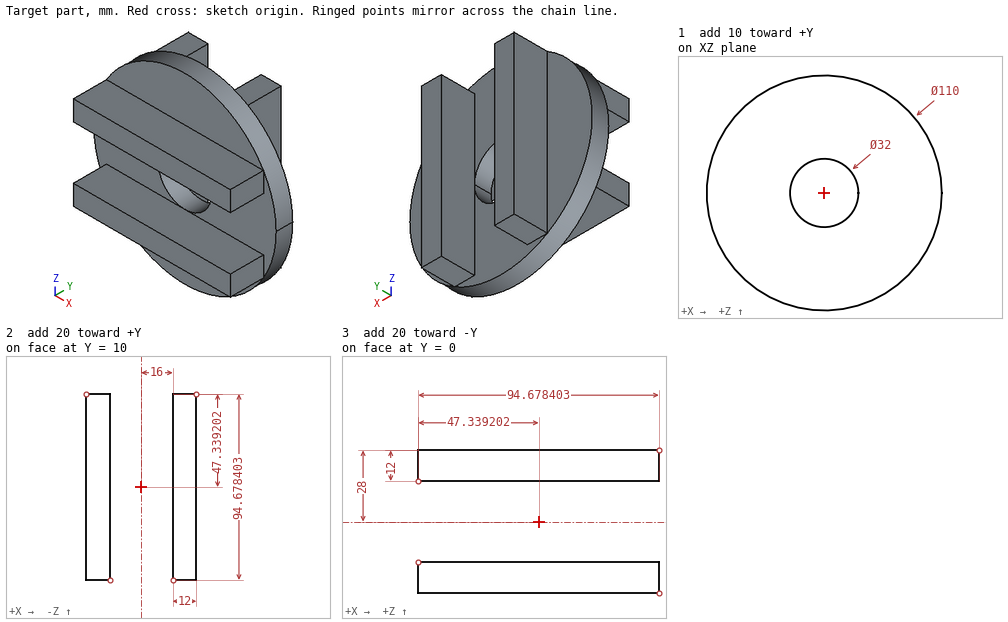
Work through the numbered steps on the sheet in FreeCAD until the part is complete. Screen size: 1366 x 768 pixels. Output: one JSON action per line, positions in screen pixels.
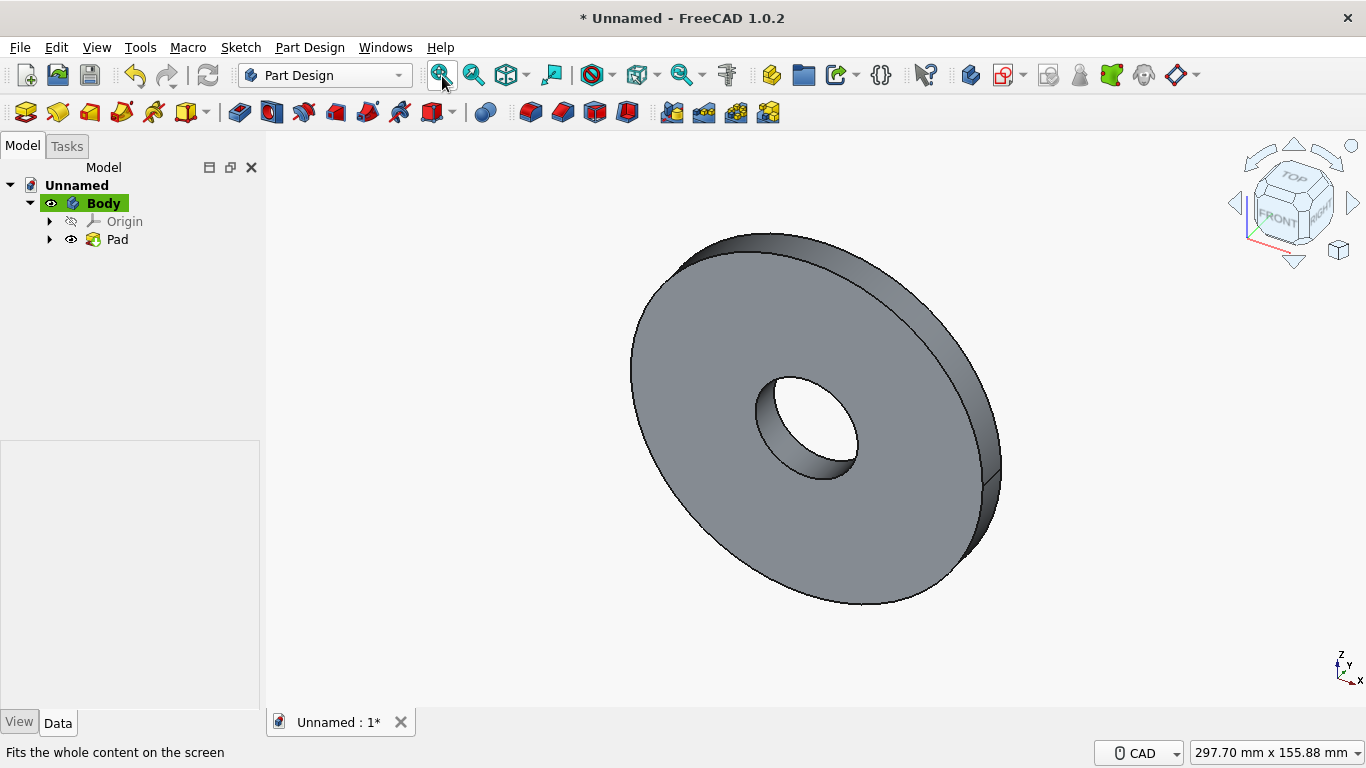
{"action": "key", "text": "4"}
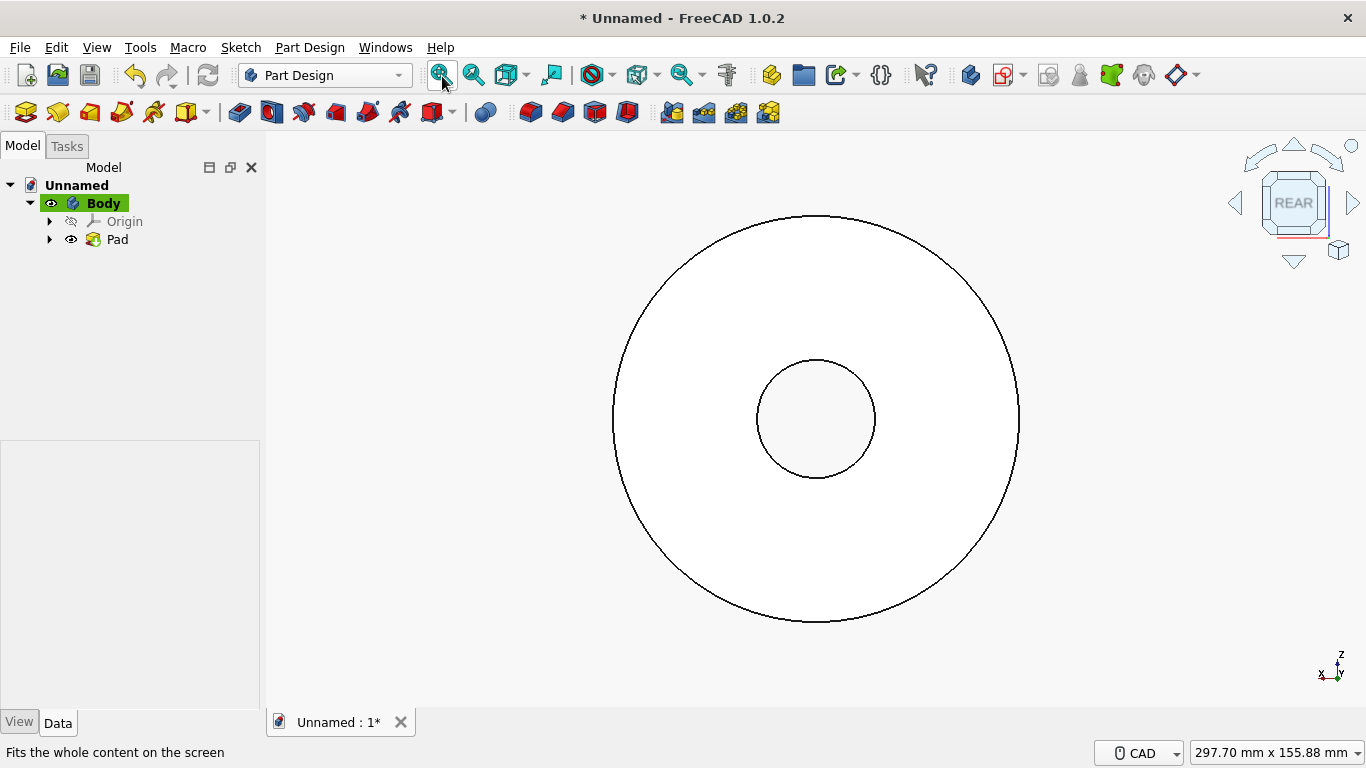
{"action": "left_click", "coordinate": [874, 302]}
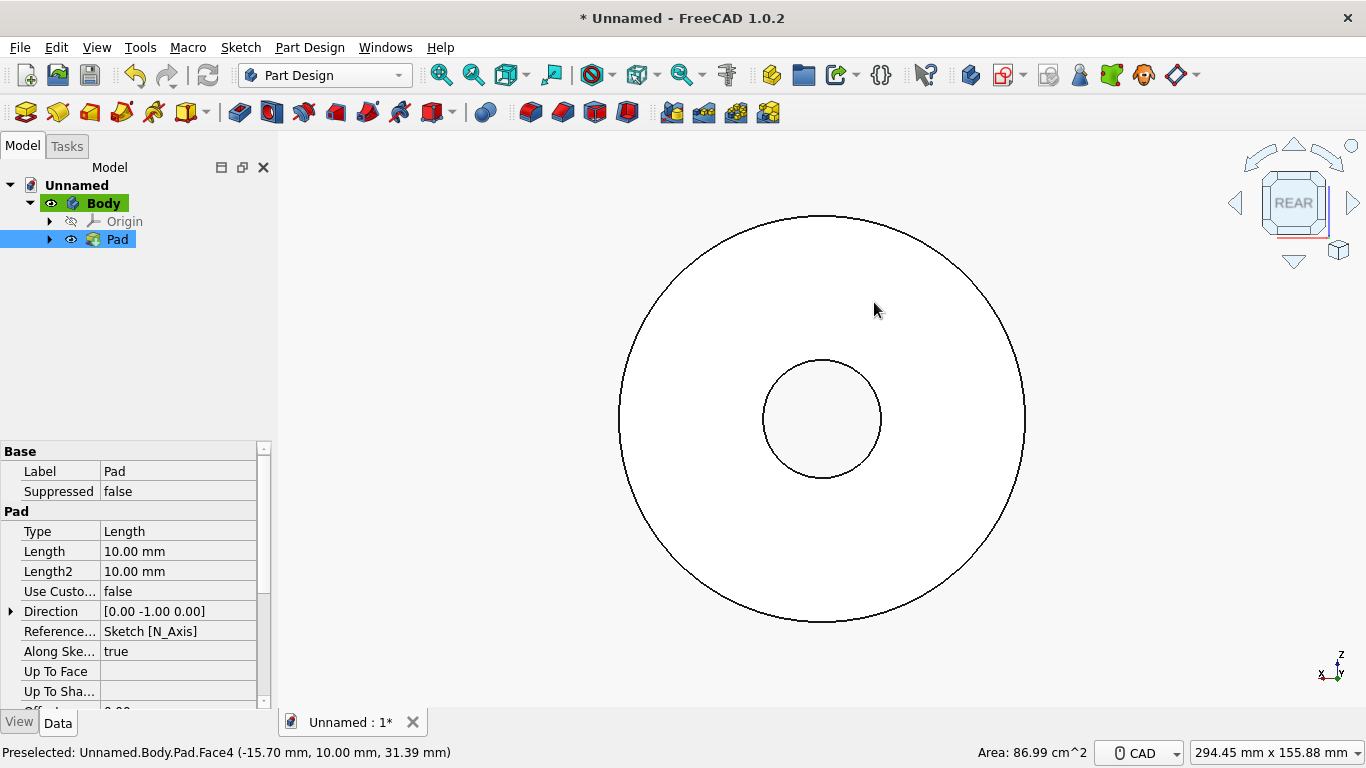
{"action": "left_click", "coordinate": [1004, 76]}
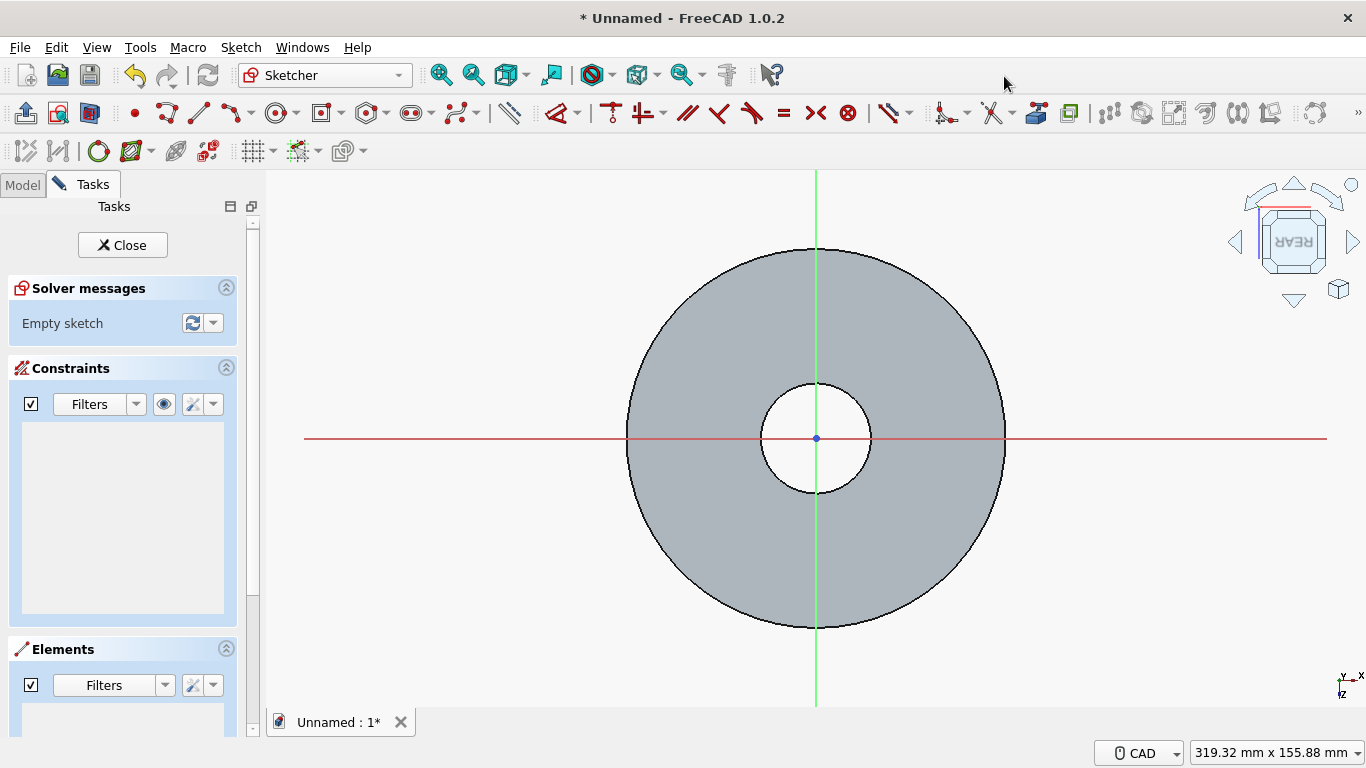
{"action": "key", "text": "g r"}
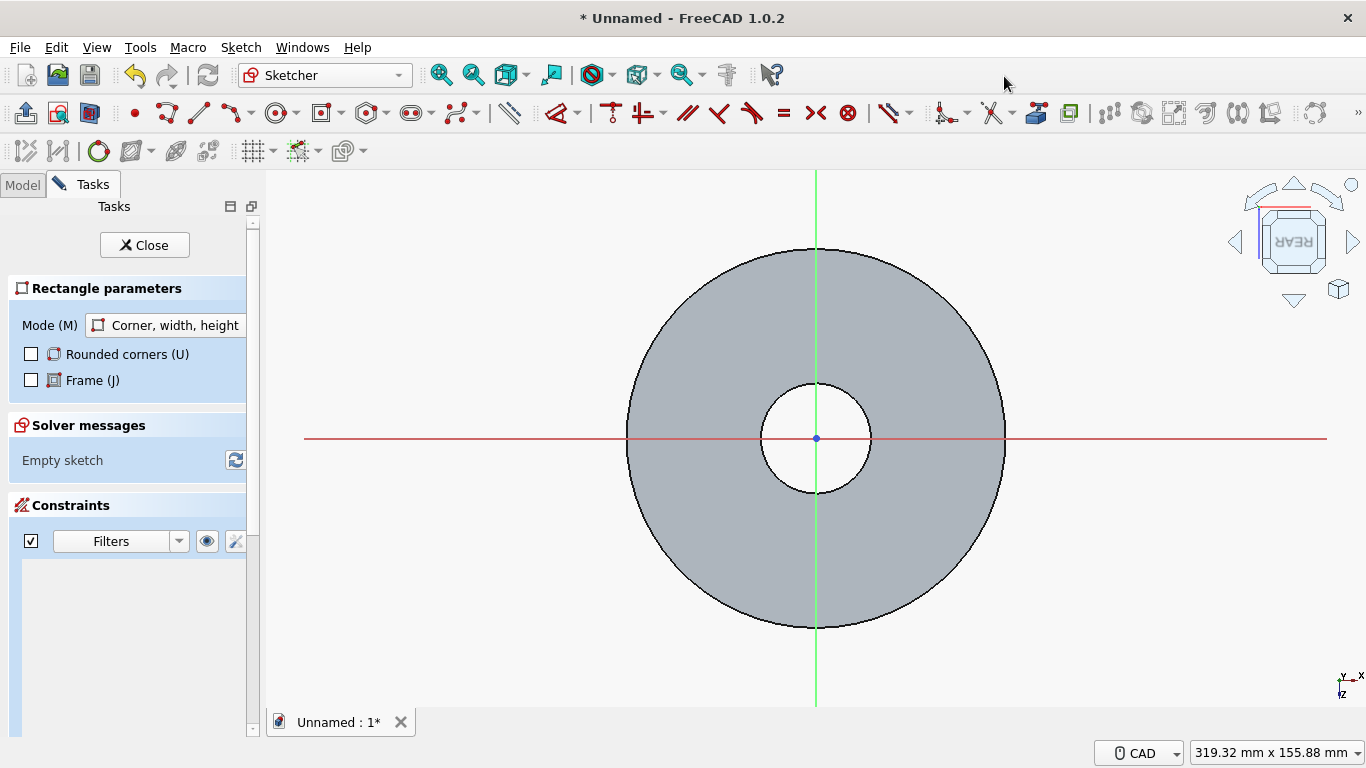
{"action": "left_click", "coordinate": [871, 275]}
{"action": "left_click", "coordinate": [912, 602]}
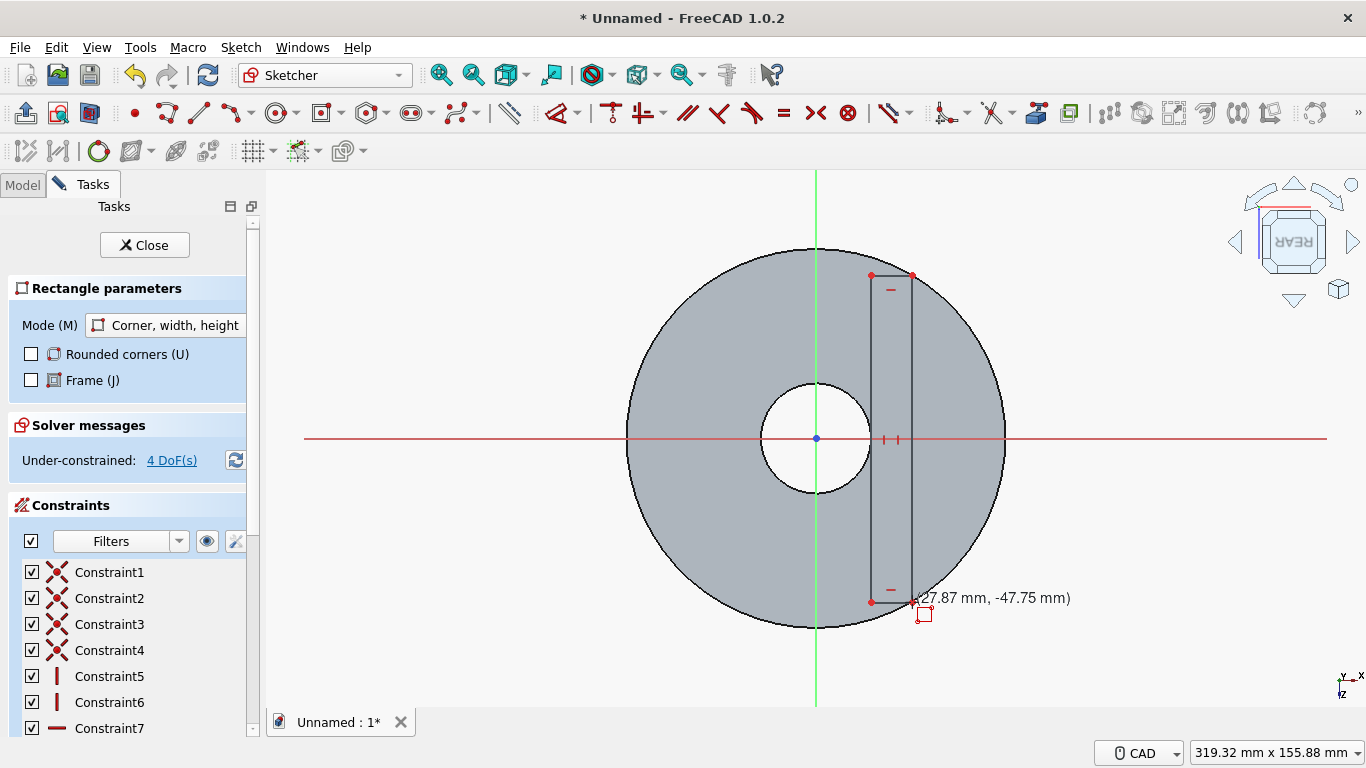
{"action": "left_click", "coordinate": [720, 275]}
{"action": "left_click", "coordinate": [761, 602]}
{"action": "key", "text": "Escape"}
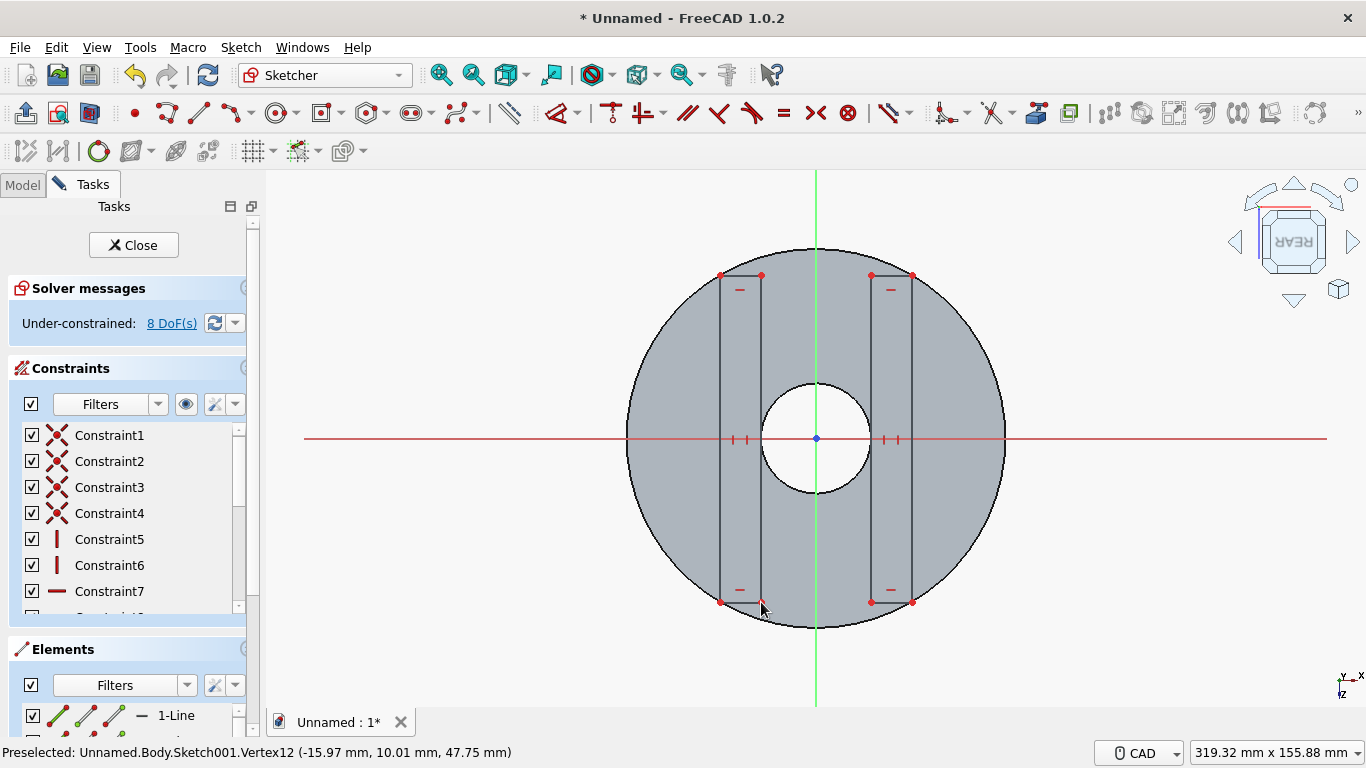
{"action": "left_click", "coordinate": [912, 276]}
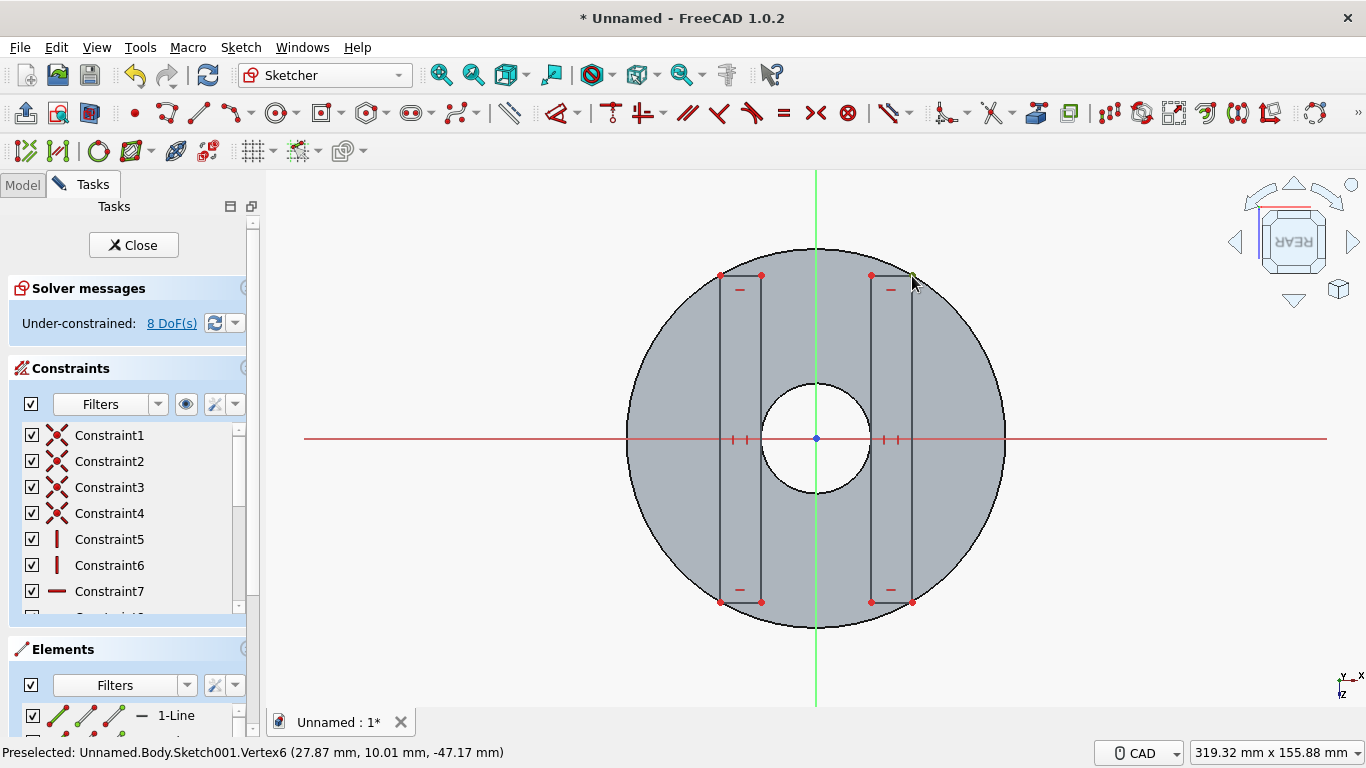
{"action": "left_click", "coordinate": [720, 276]}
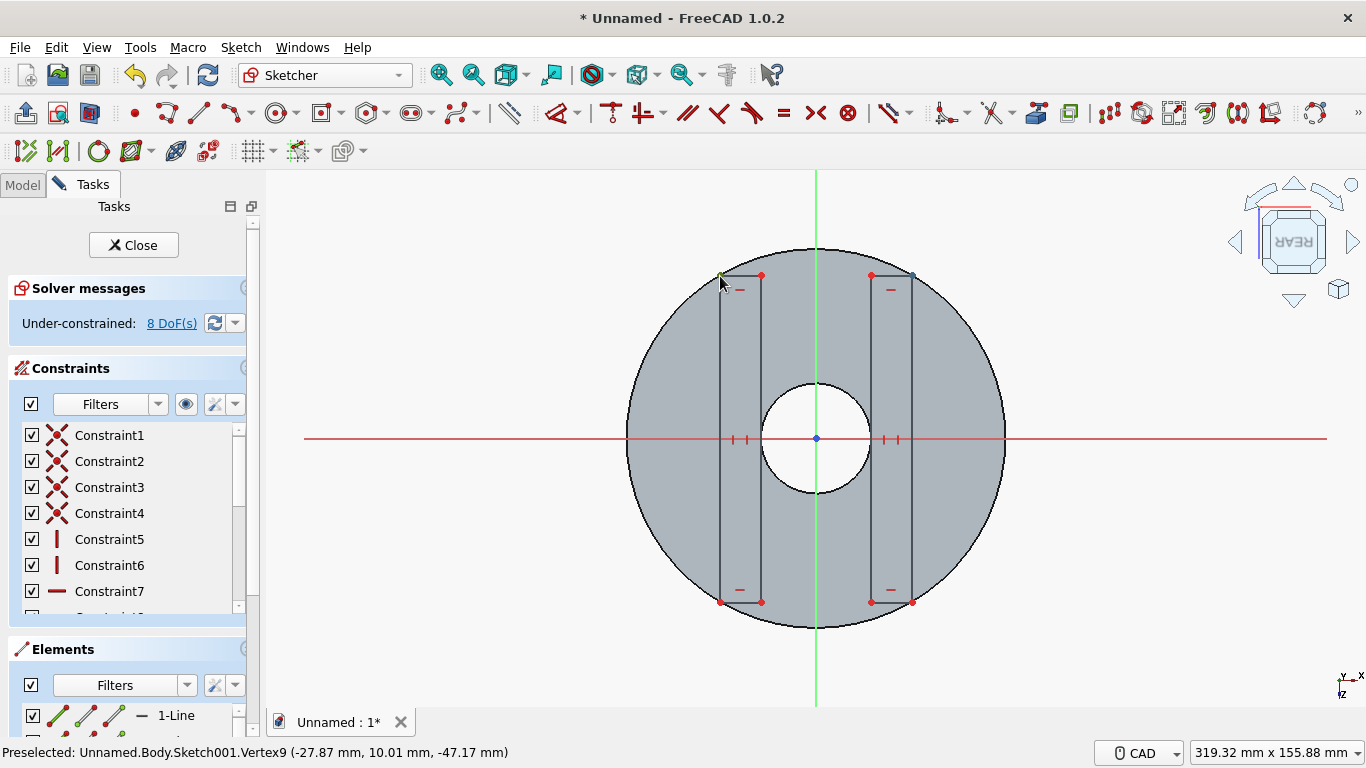
{"action": "left_click", "coordinate": [816, 645]}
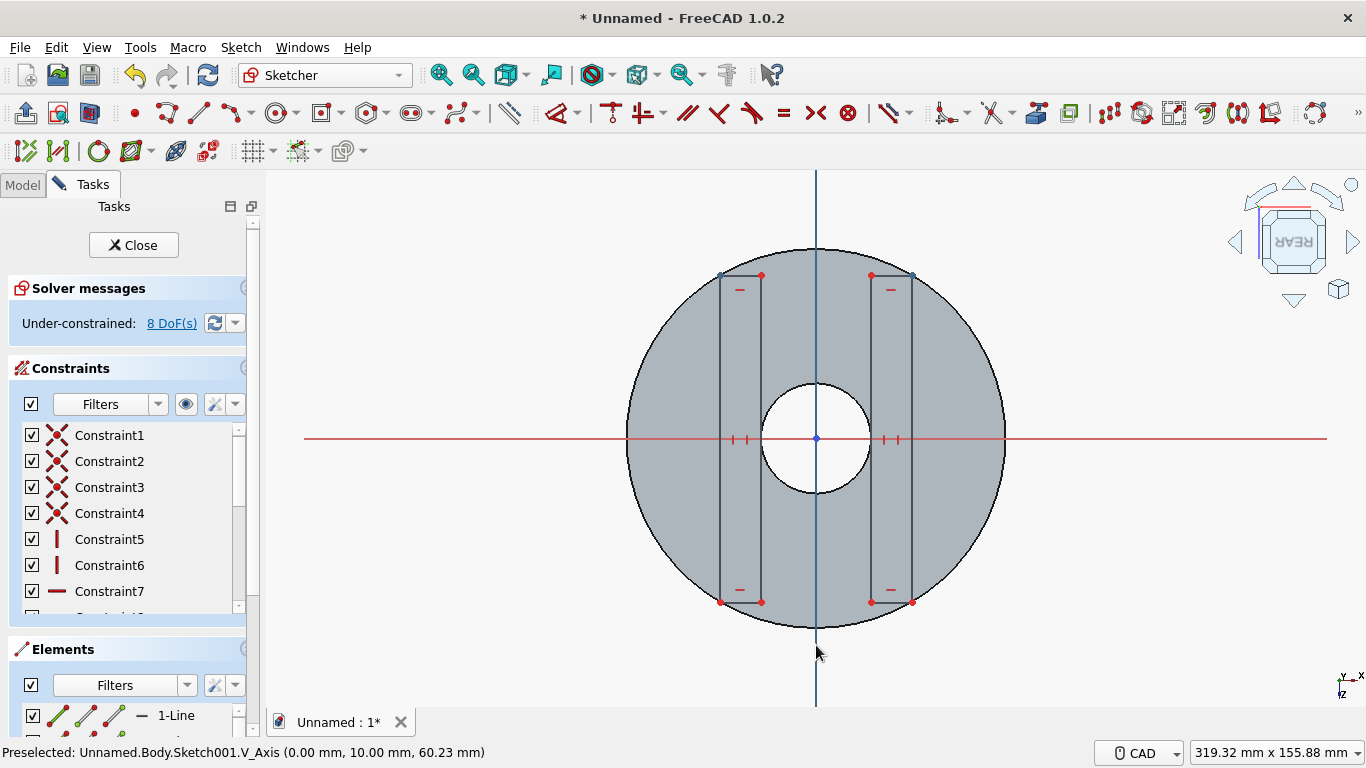
{"action": "key", "text": "s"}